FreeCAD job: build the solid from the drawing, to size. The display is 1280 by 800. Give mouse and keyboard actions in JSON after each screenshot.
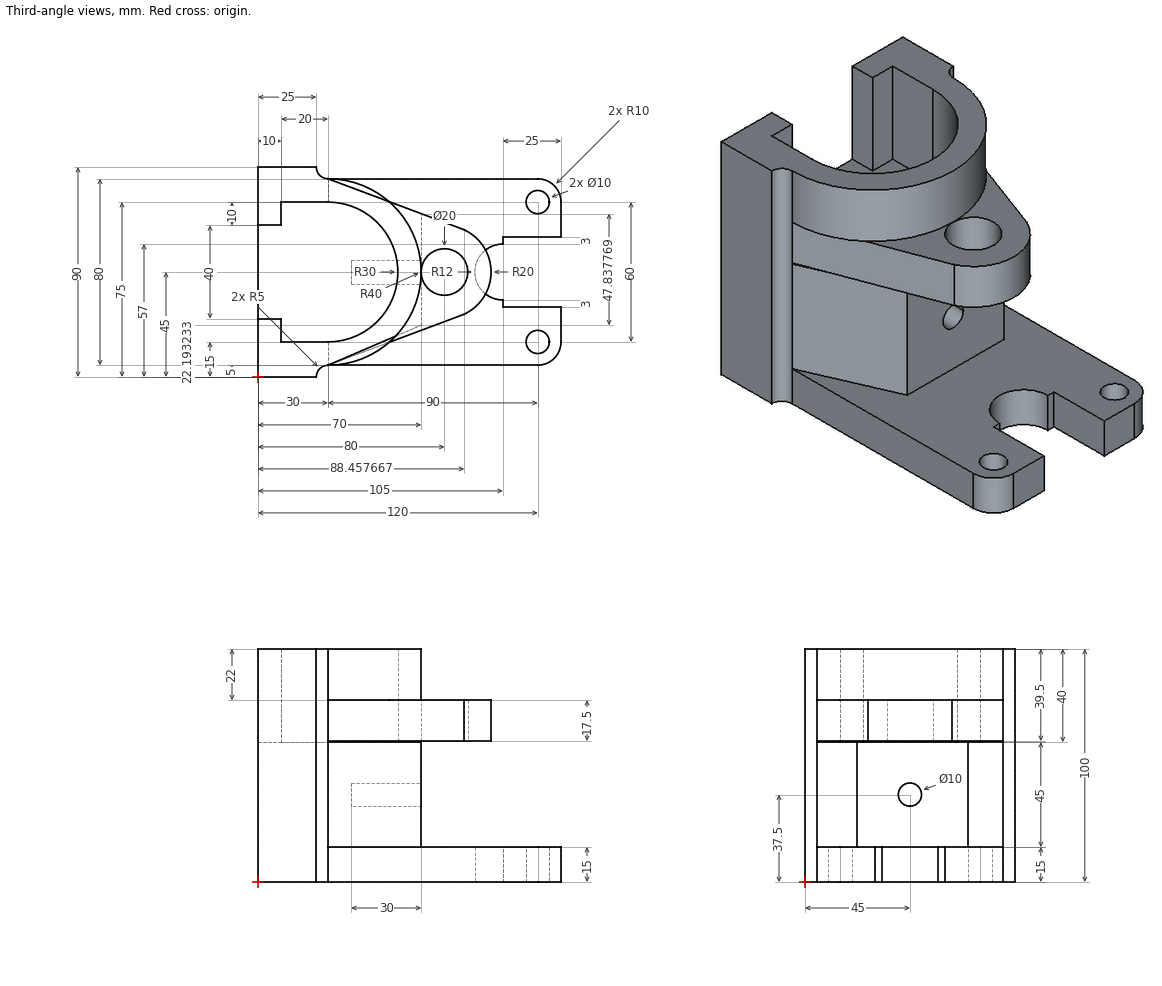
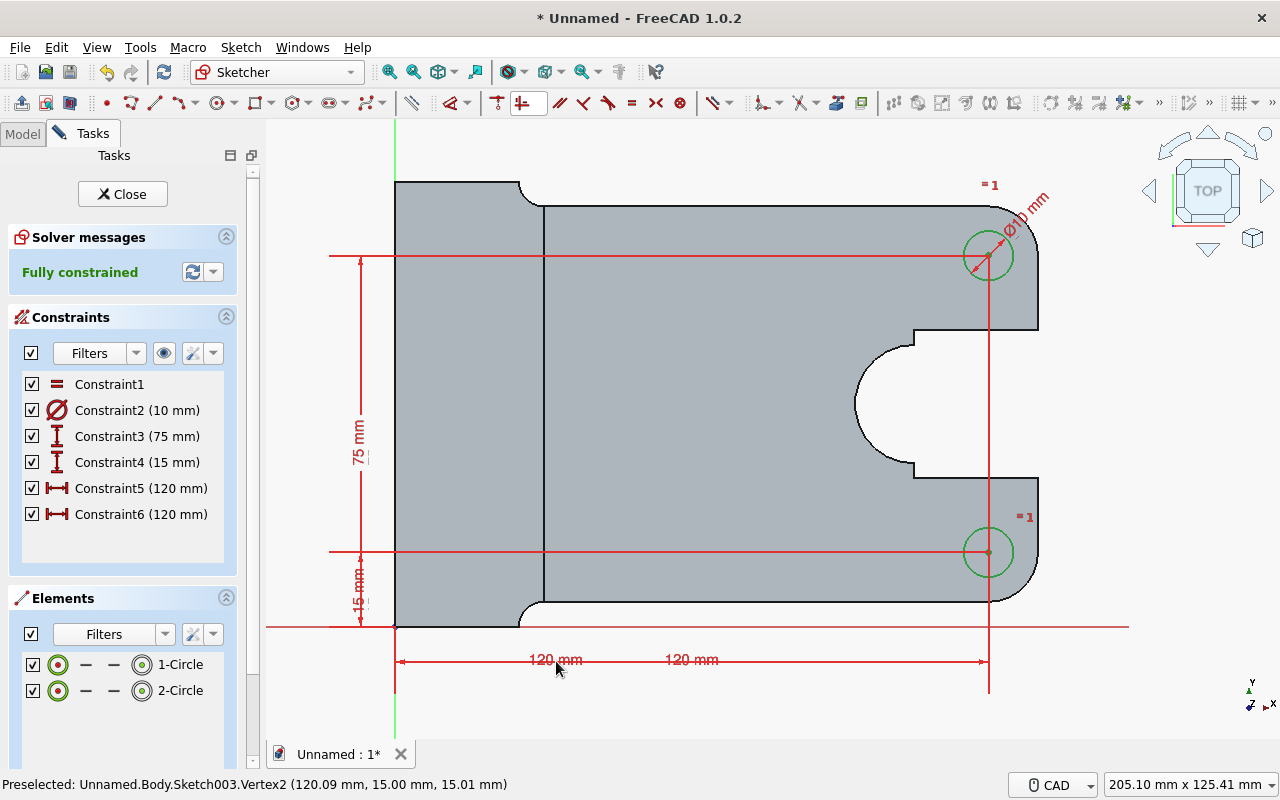
{"action": "left_click", "coordinate": [123, 194]}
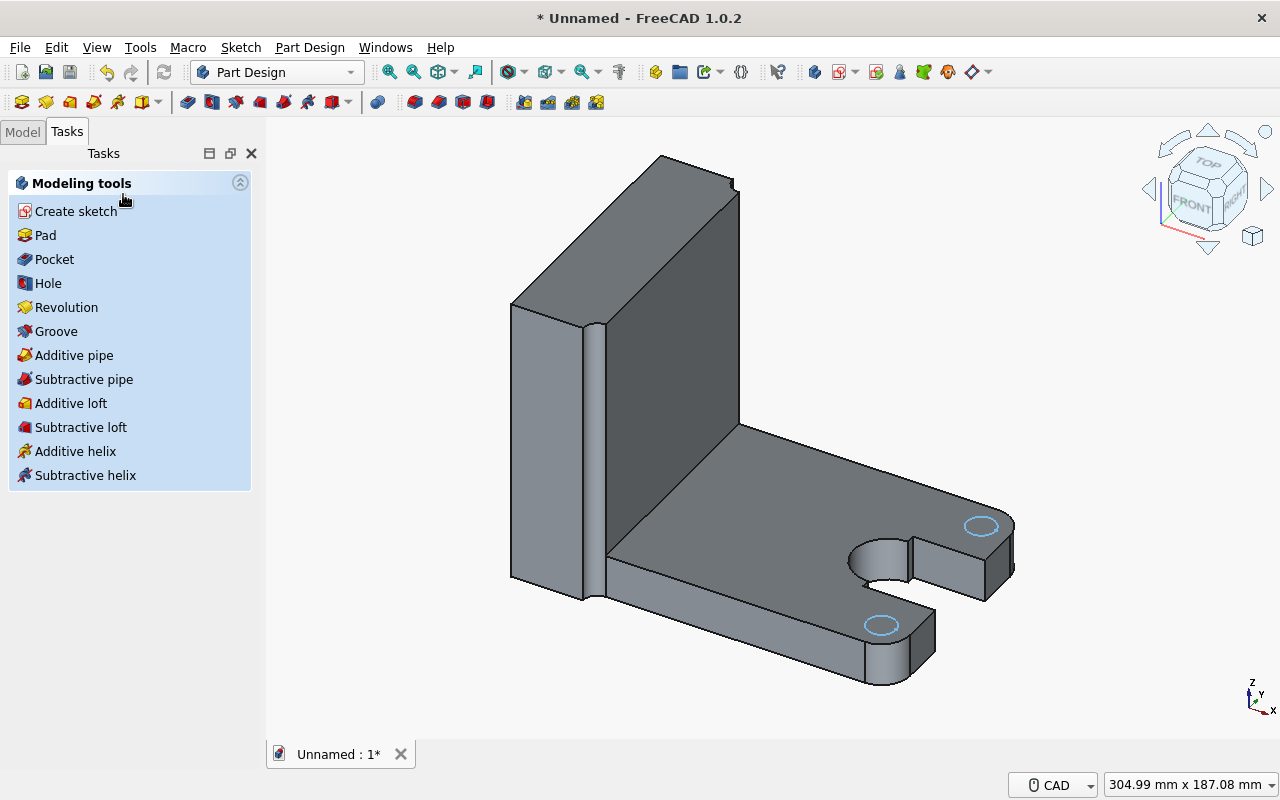
{"action": "left_click", "coordinate": [188, 102]}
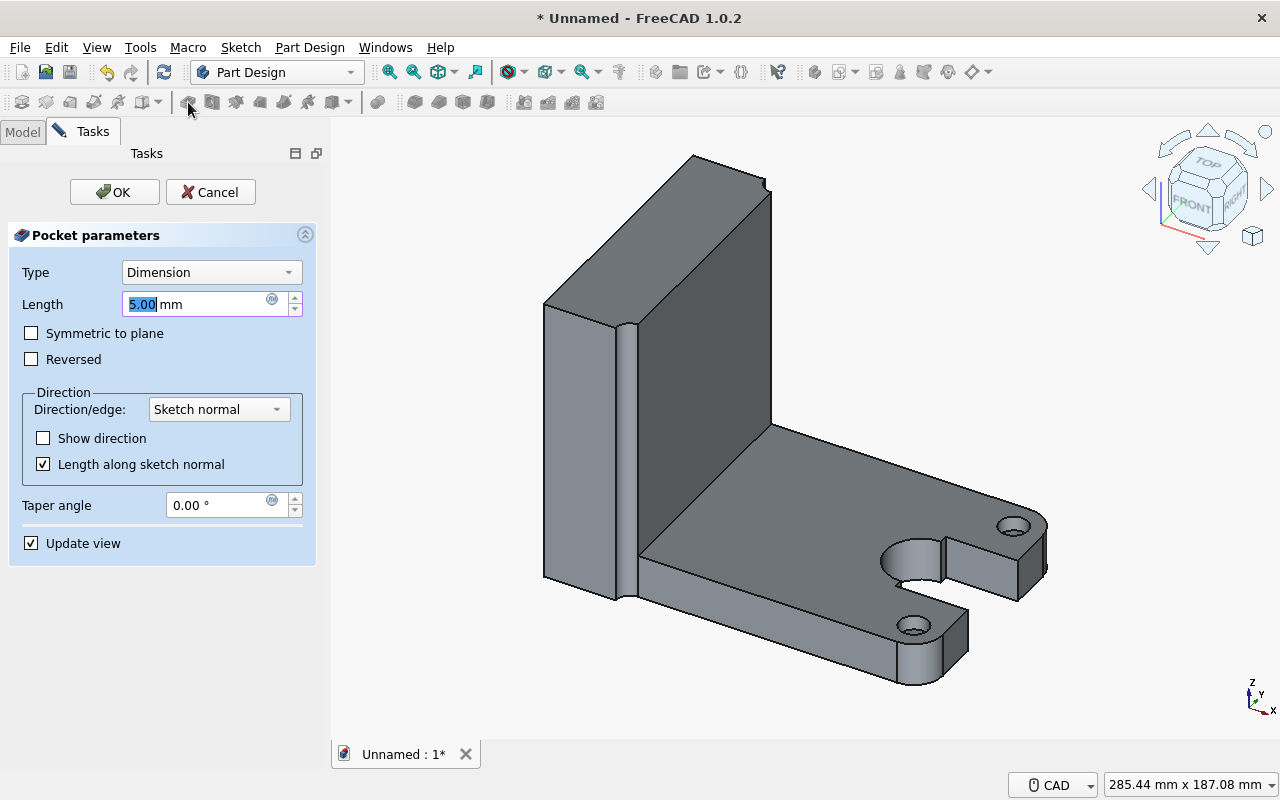
{"action": "type", "text": "15"}
{"action": "key", "text": "Tab"}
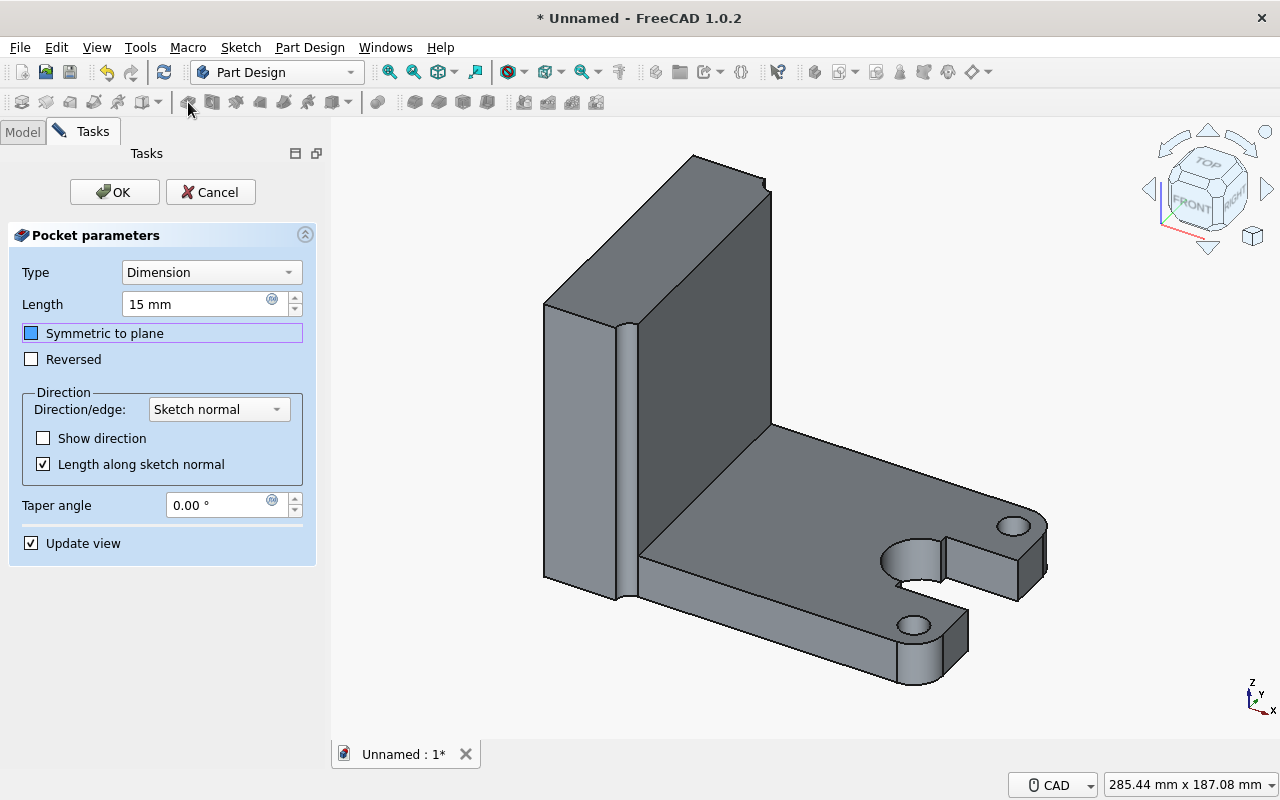
{"action": "left_click", "coordinate": [115, 192]}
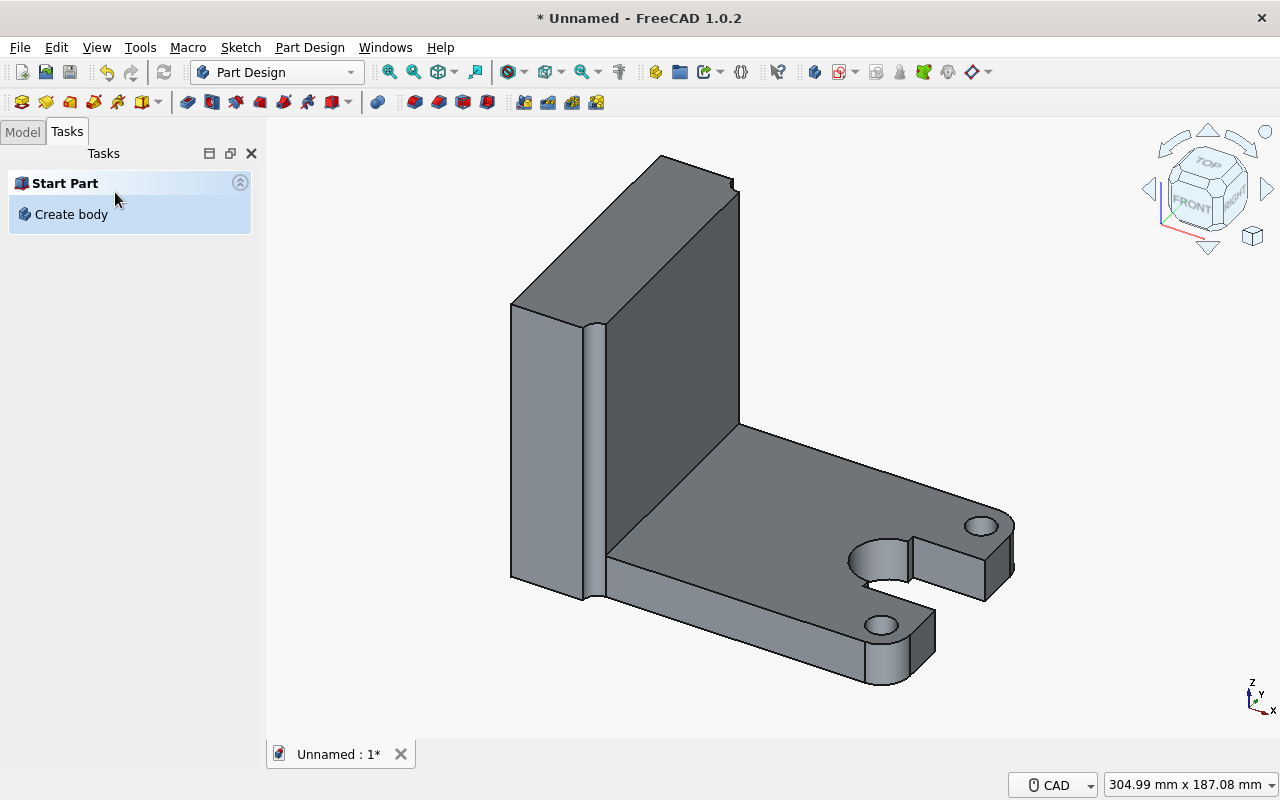
{"action": "left_click", "coordinate": [672, 201]}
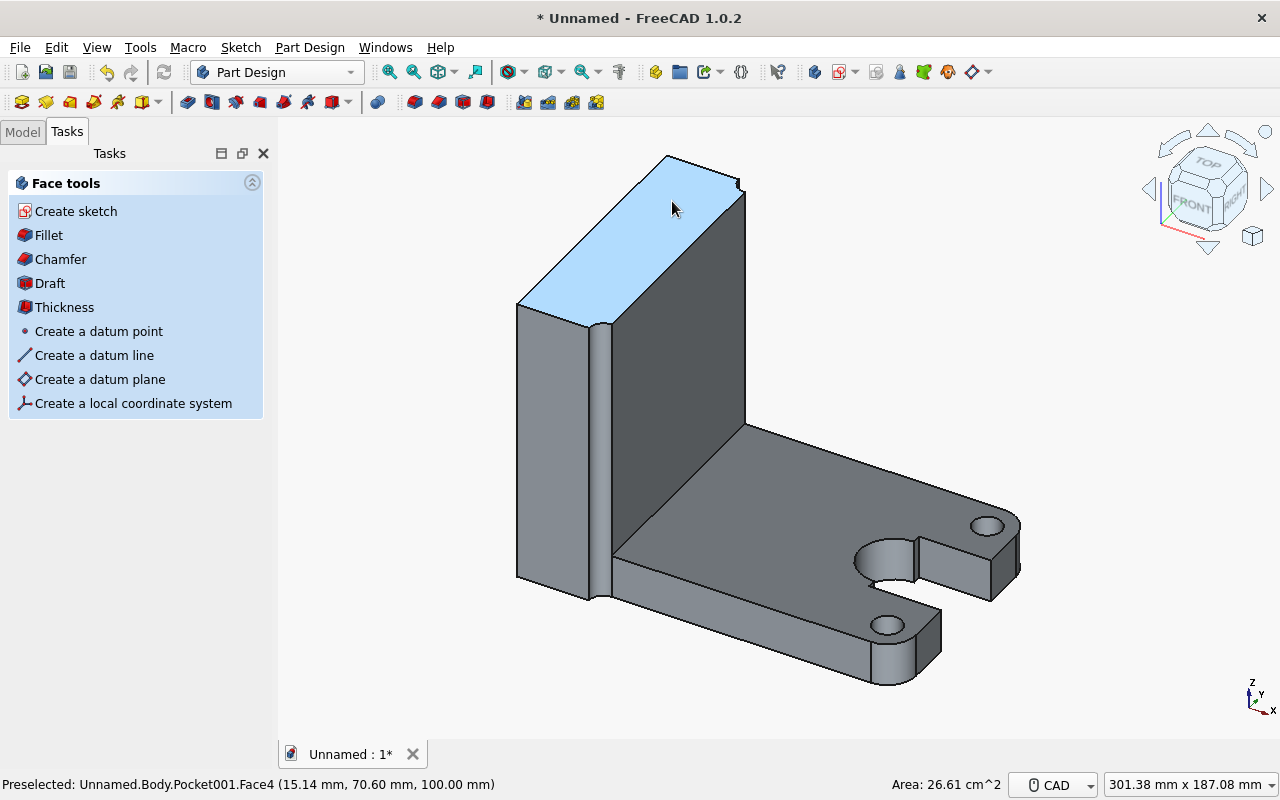
{"action": "left_click", "coordinate": [840, 72]}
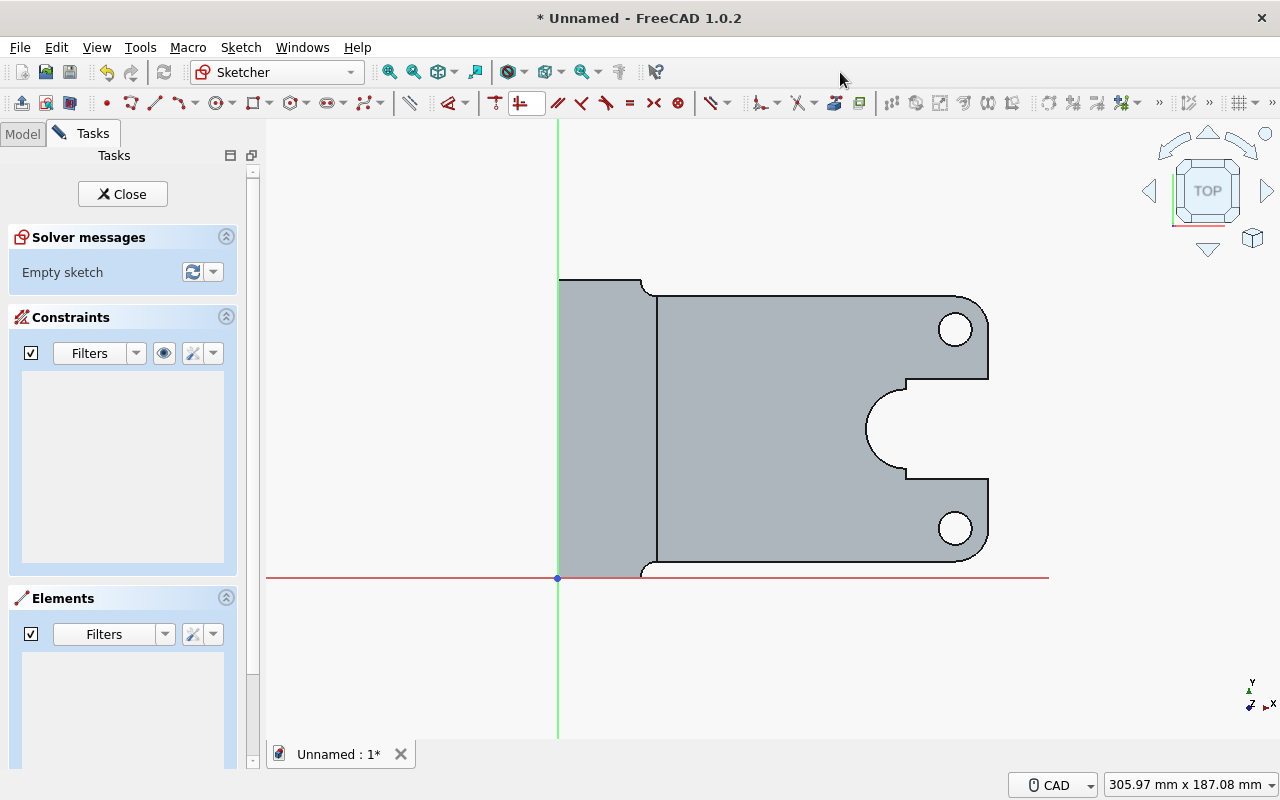
{"action": "scroll", "coordinate": [761, 454], "scroll_direction": "up", "scroll_amount": 2}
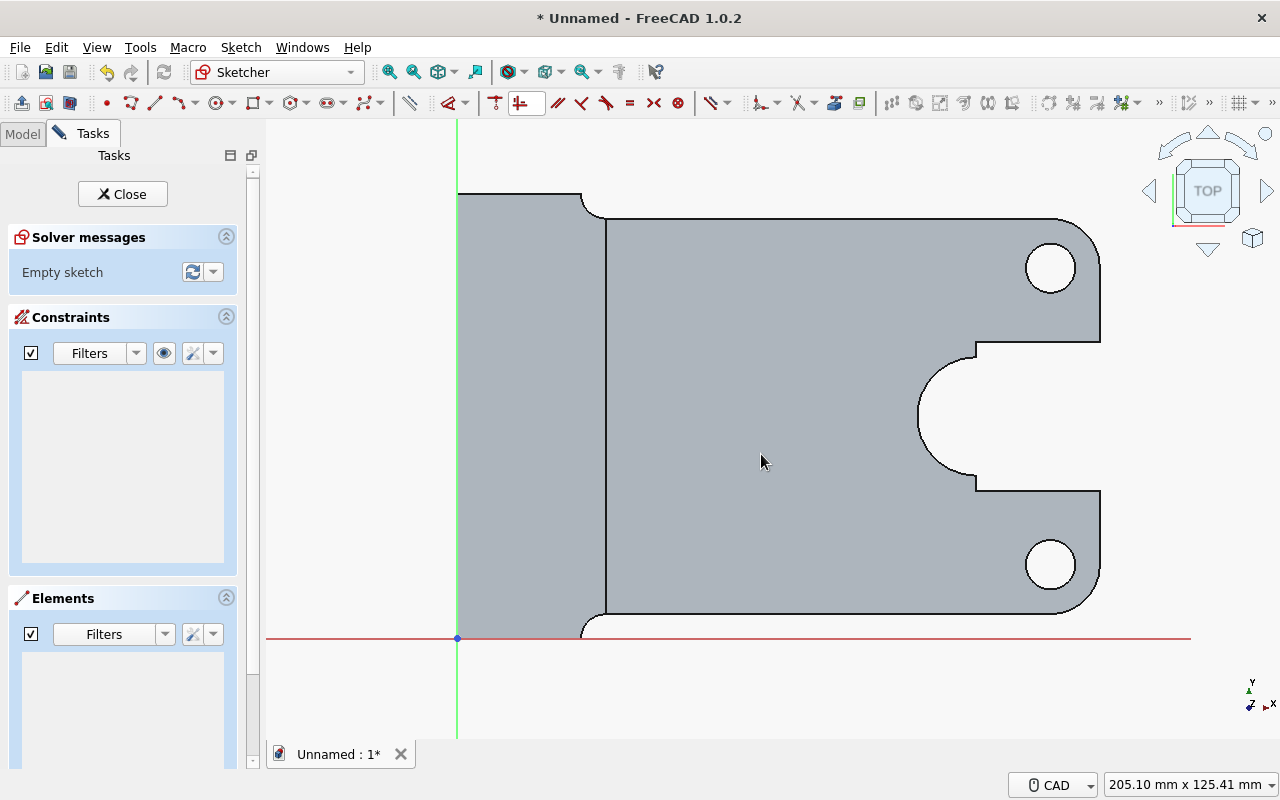
{"action": "left_click", "coordinate": [132, 104]}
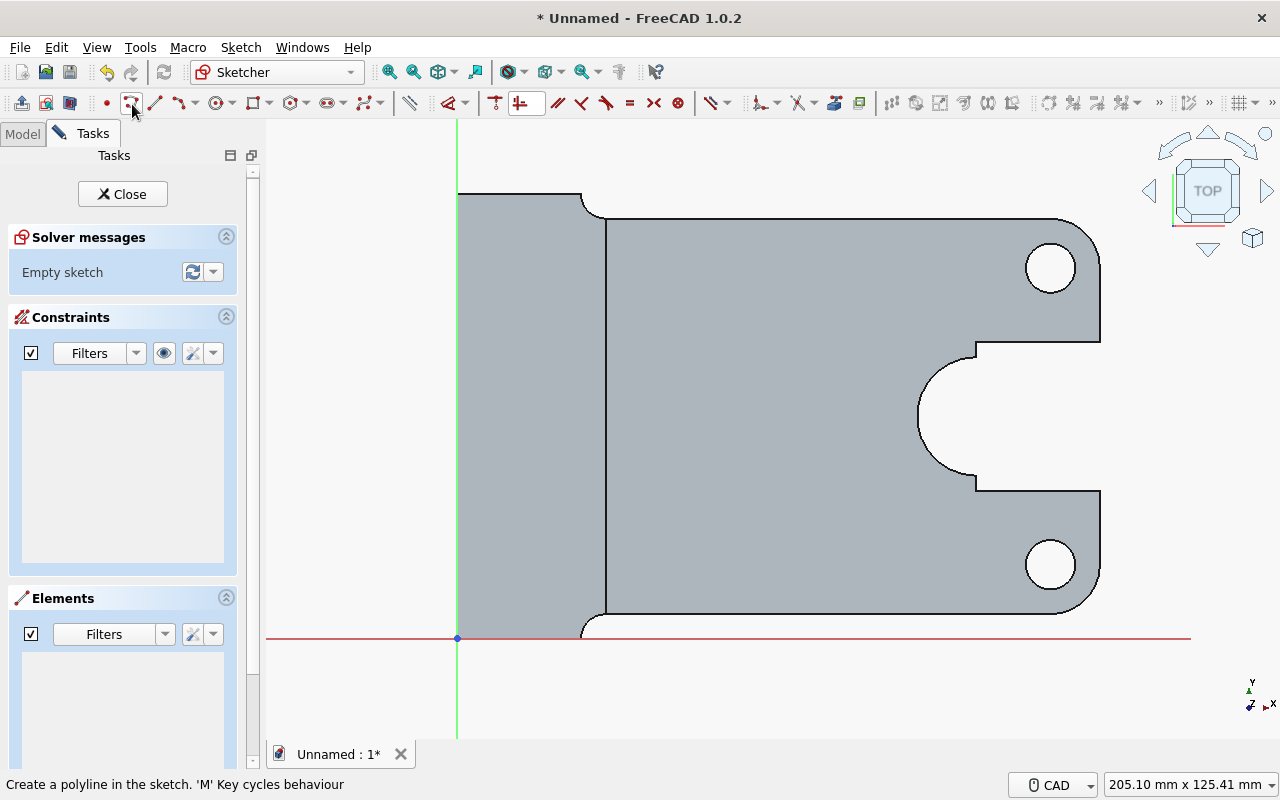
{"action": "left_click", "coordinate": [895, 327]}
{"action": "left_click", "coordinate": [606, 219]}
{"action": "left_click", "coordinate": [606, 614]}
{"action": "left_click", "coordinate": [895, 506]}
{"action": "right_click", "coordinate": [895, 506]}